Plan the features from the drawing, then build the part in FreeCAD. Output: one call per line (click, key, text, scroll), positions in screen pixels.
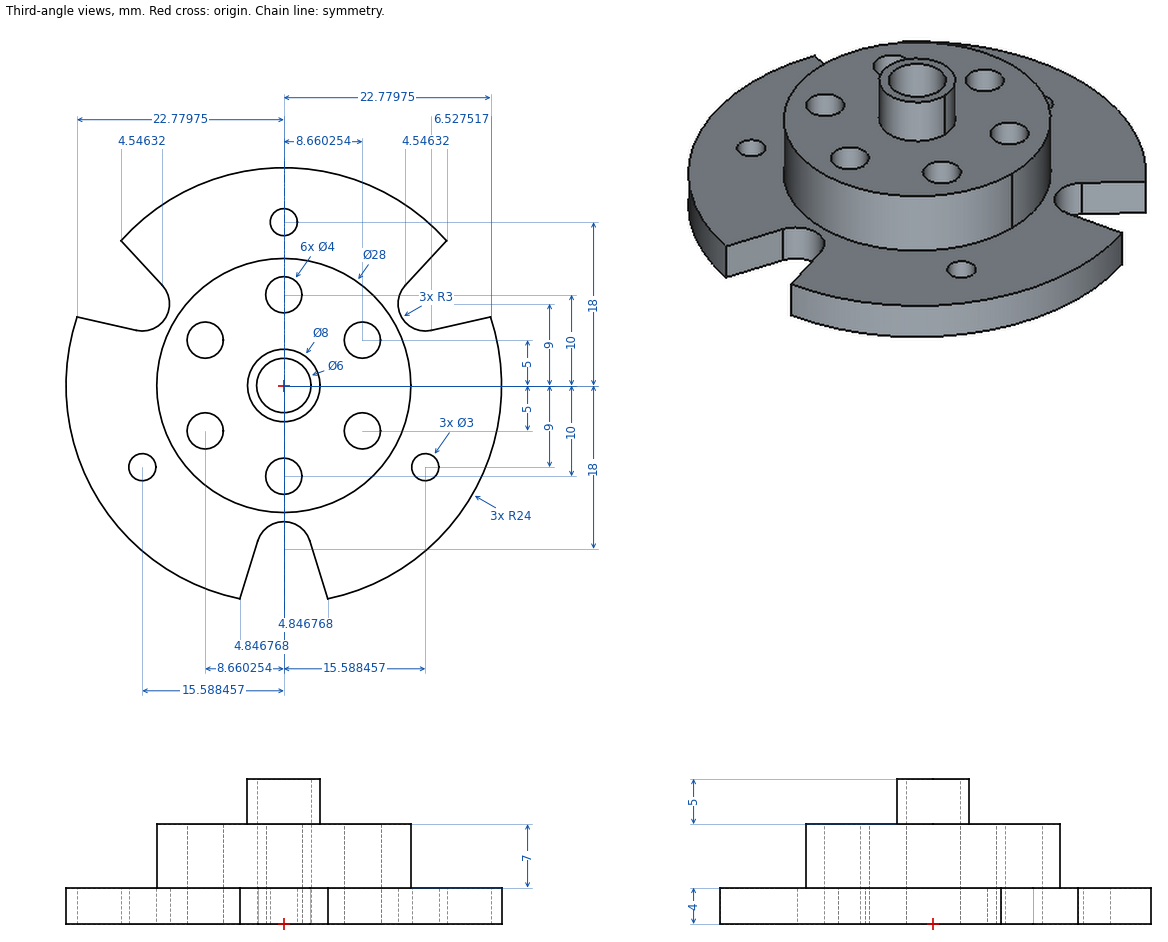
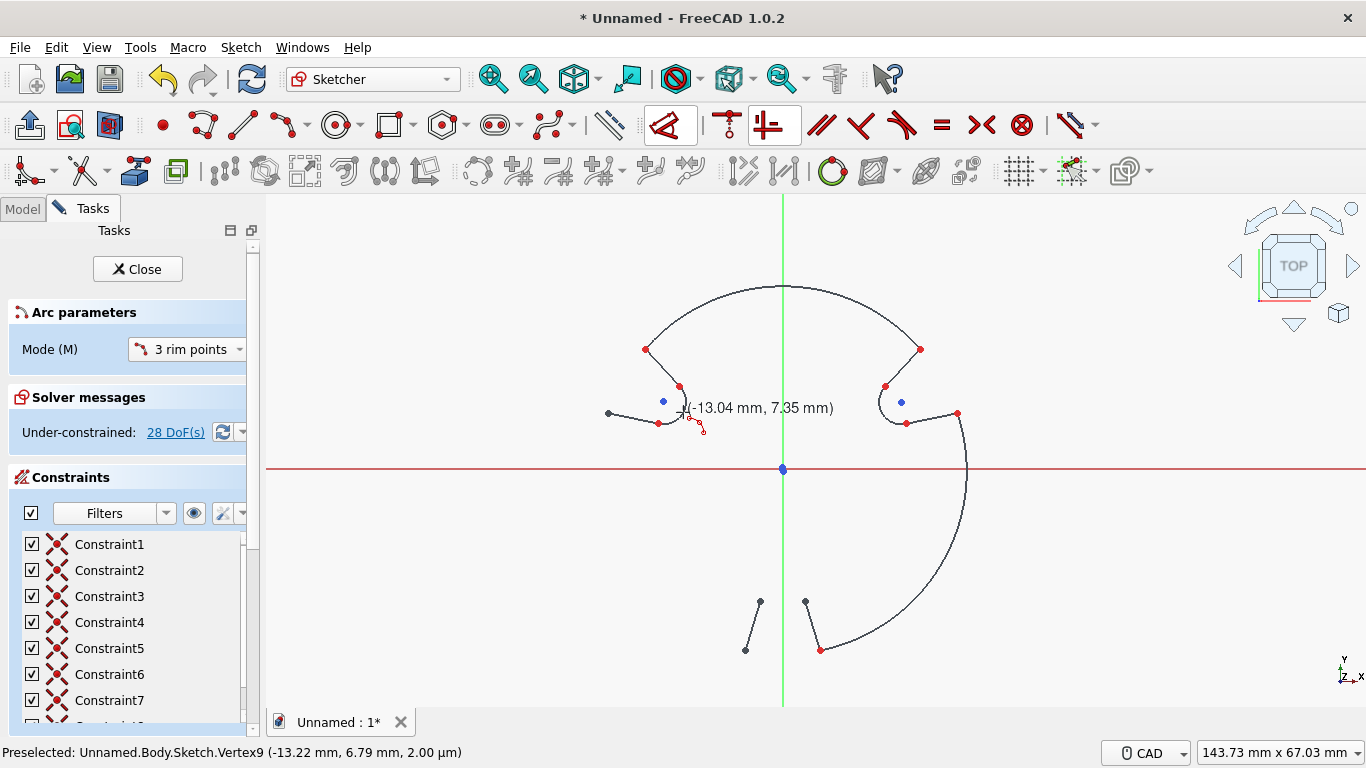
click(608, 413)
click(745, 650)
click(624, 561)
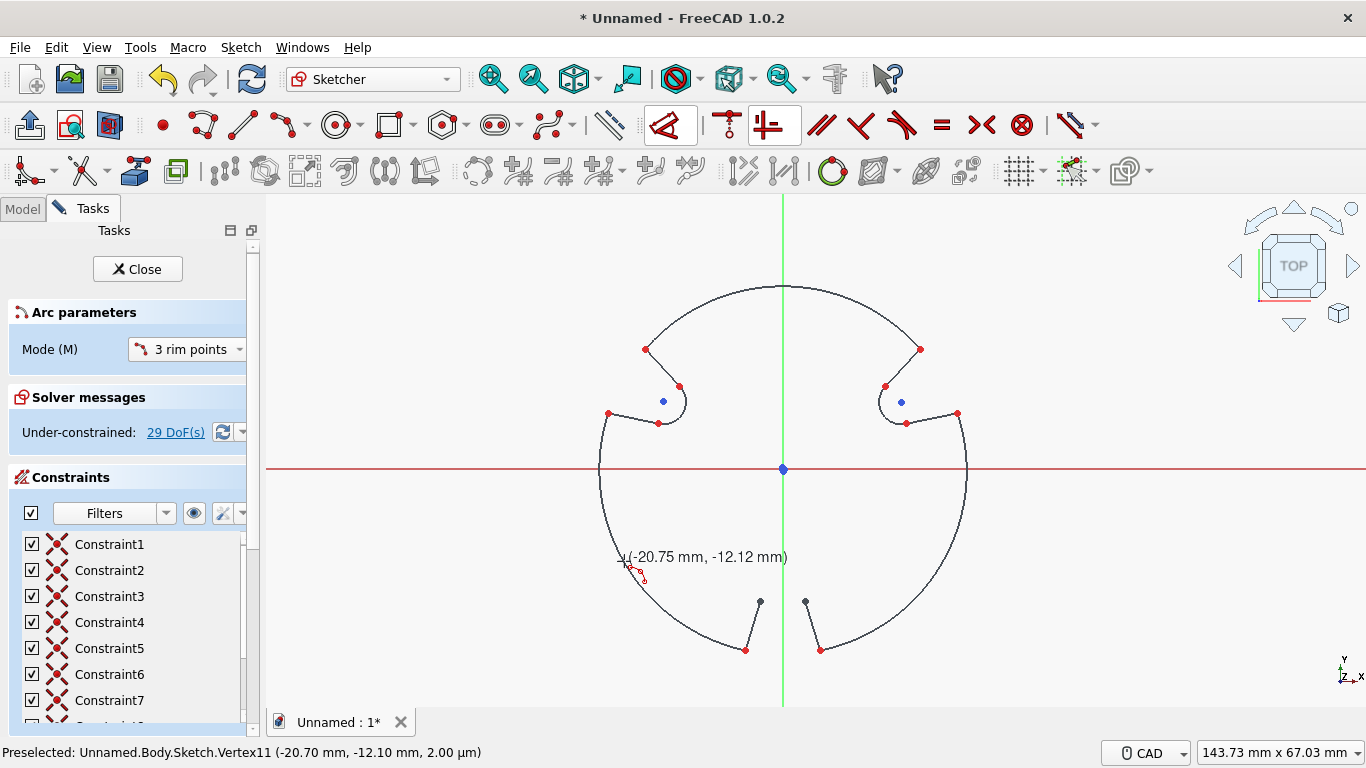
click(760, 601)
click(805, 601)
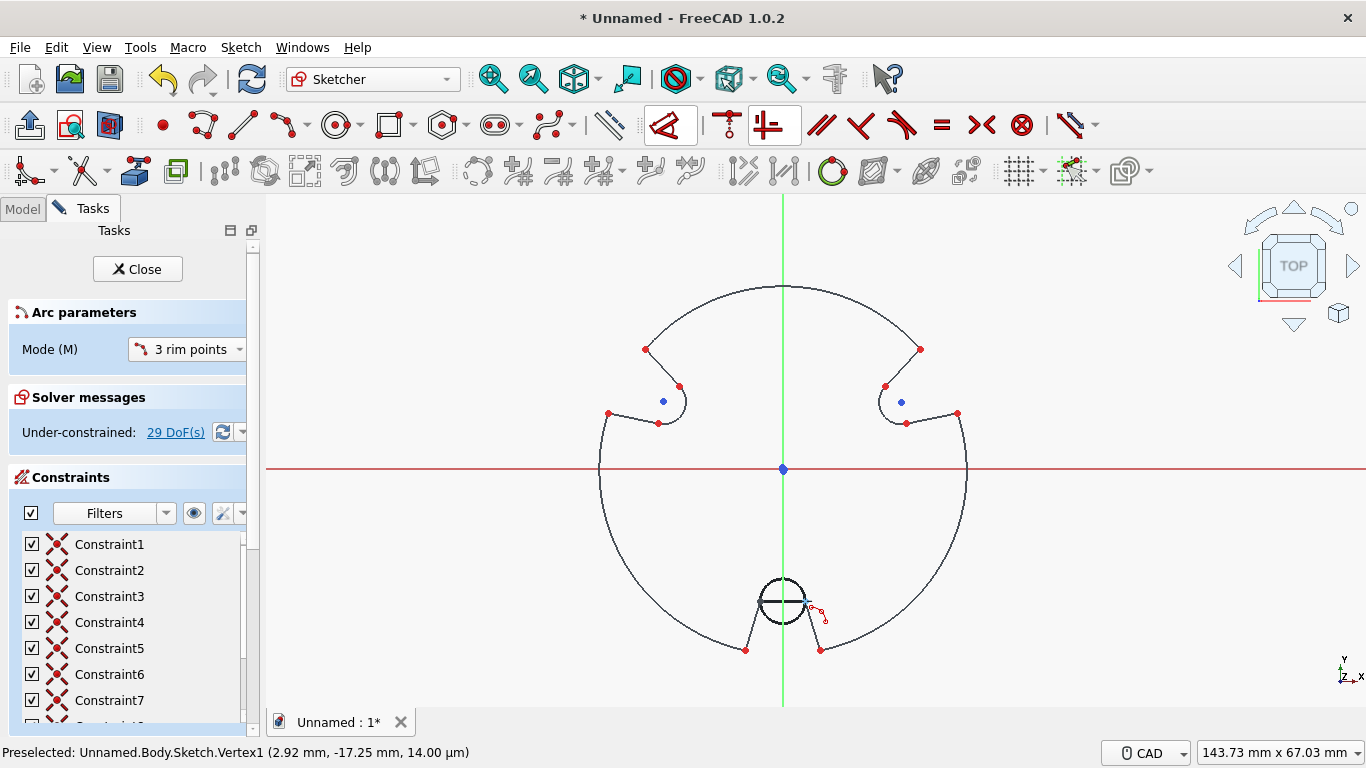
scroll(794, 587, up, 2)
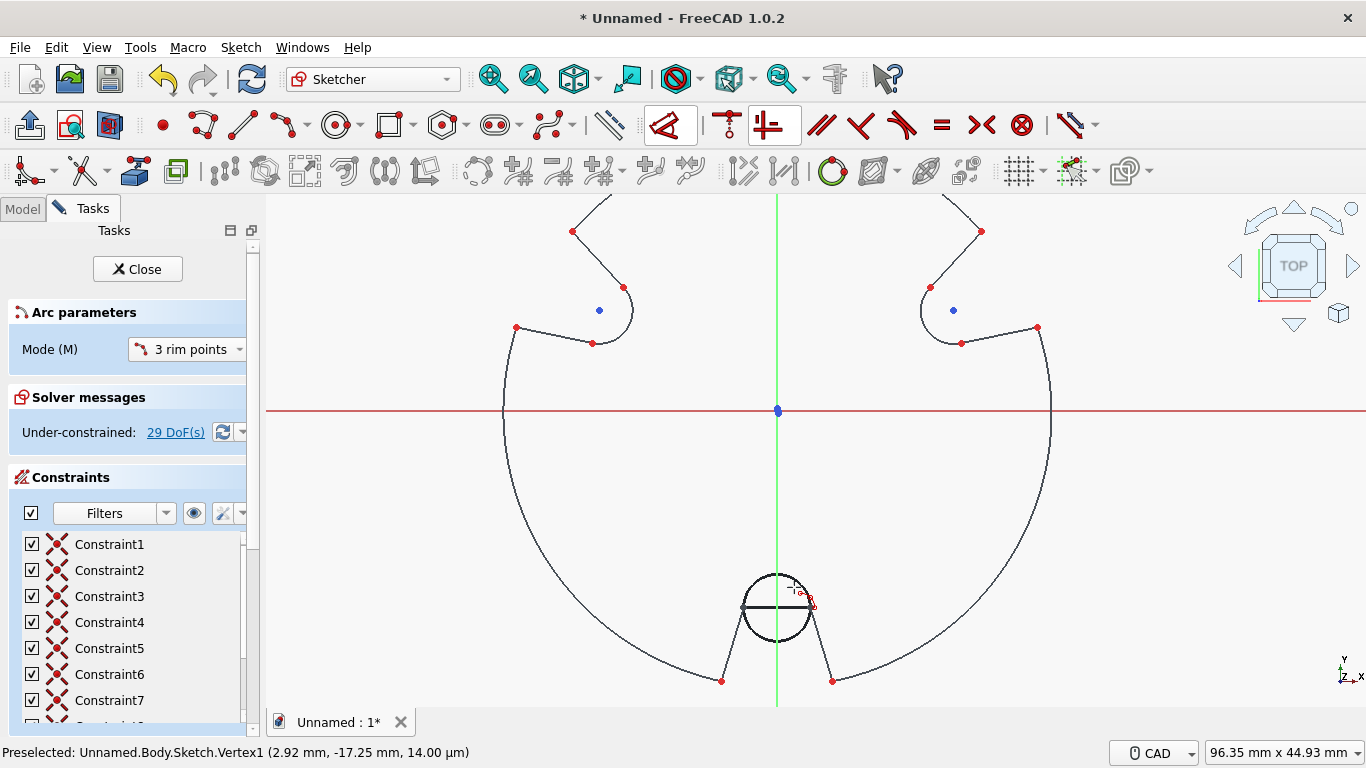
click(794, 587)
key(Escape)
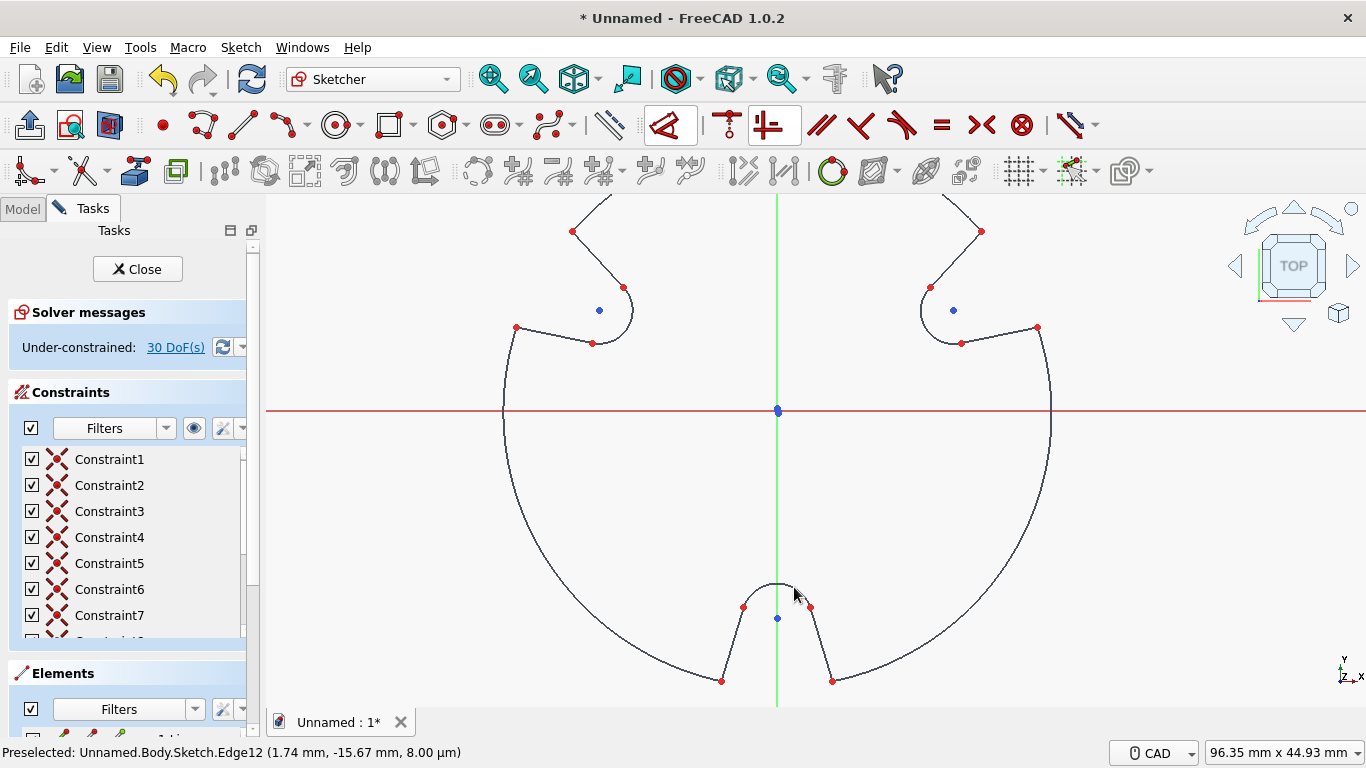
click(817, 630)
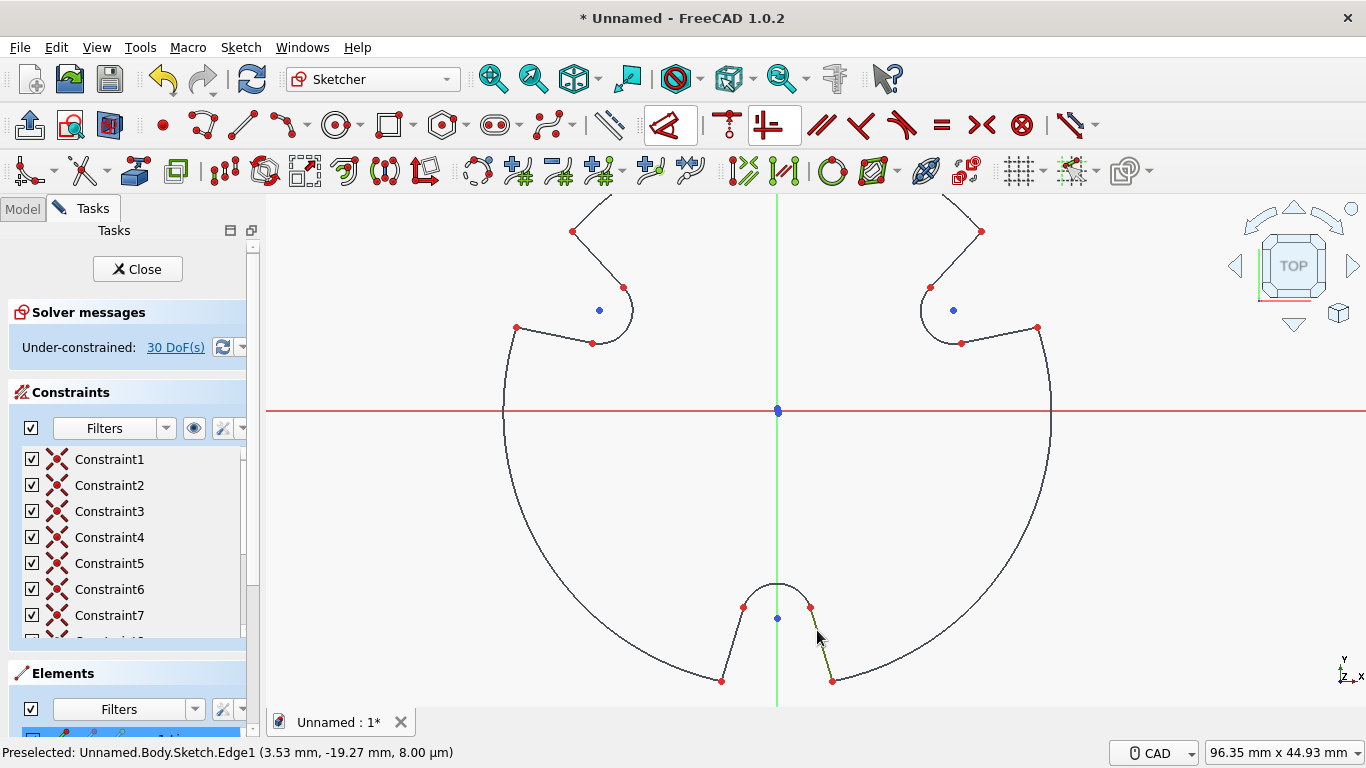
click(794, 588)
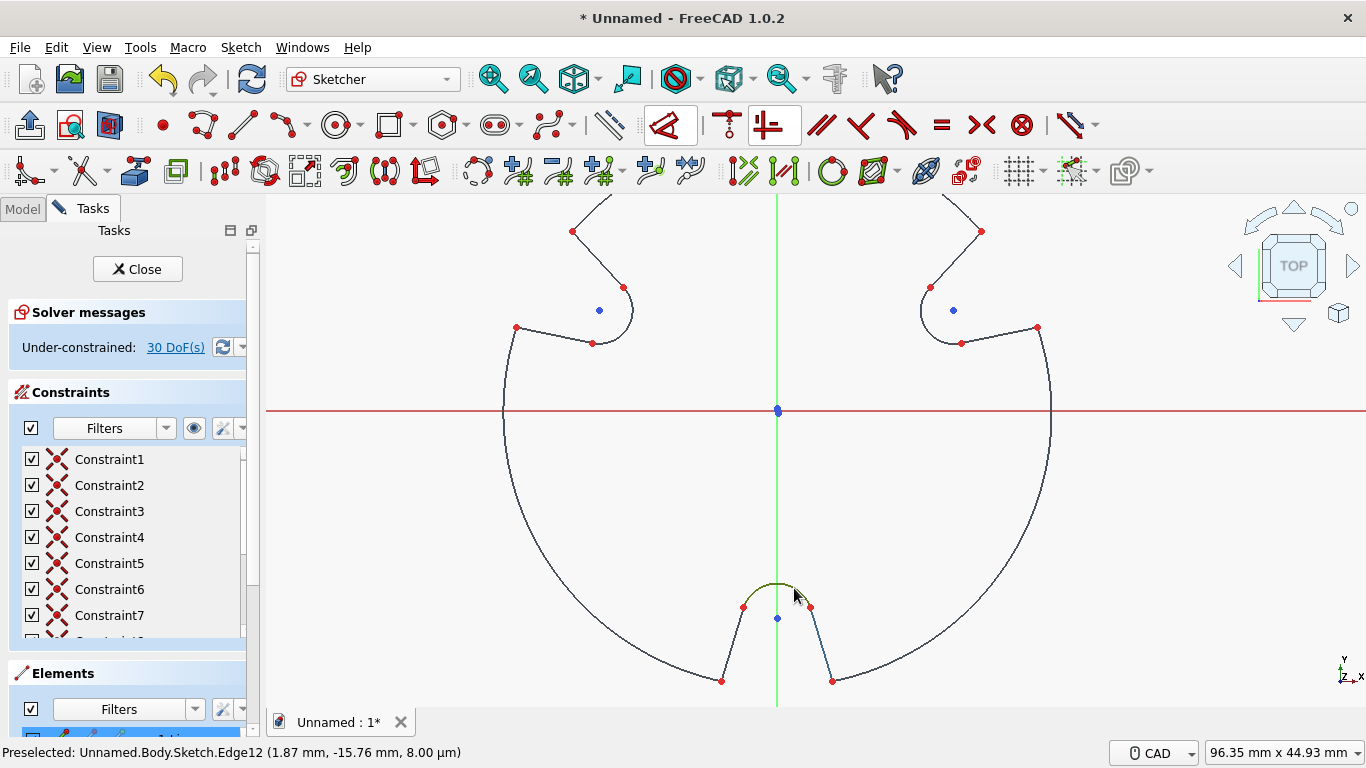
key(t)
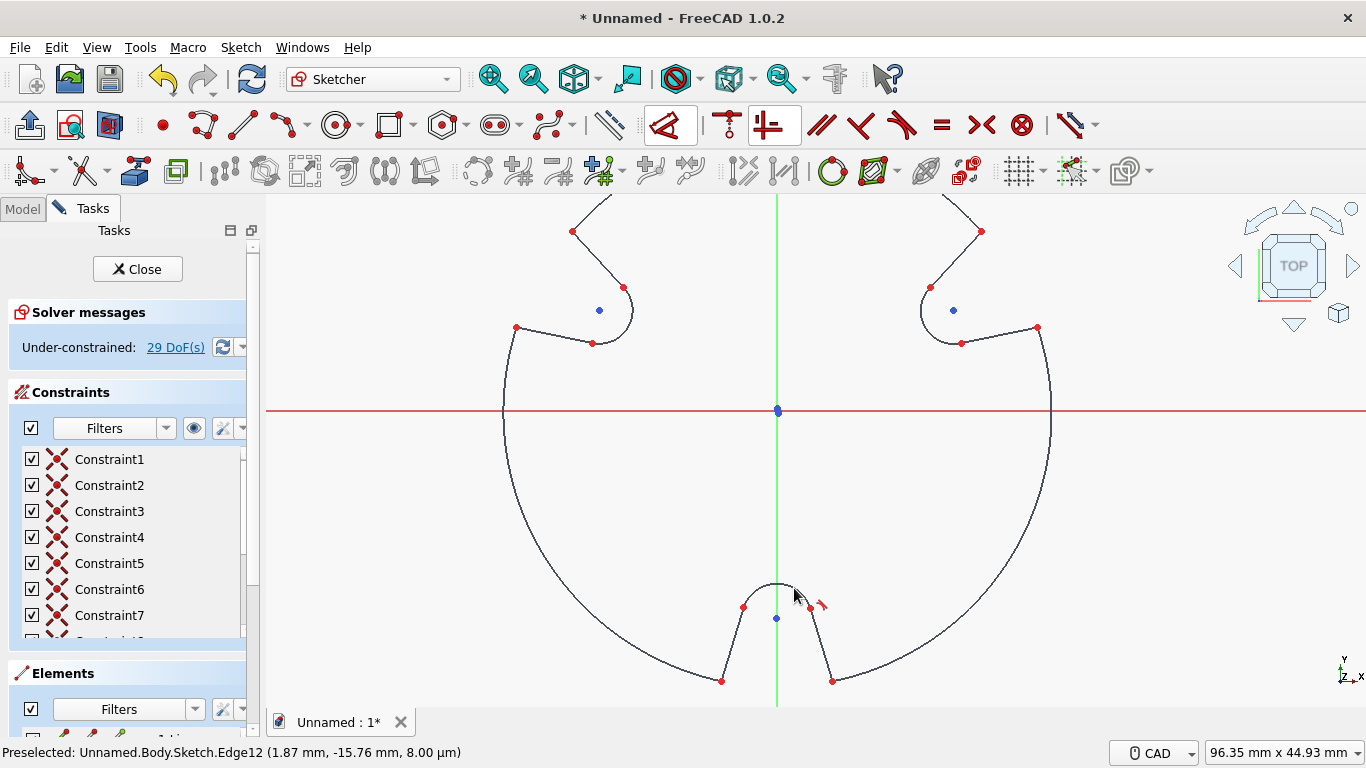
click(1015, 332)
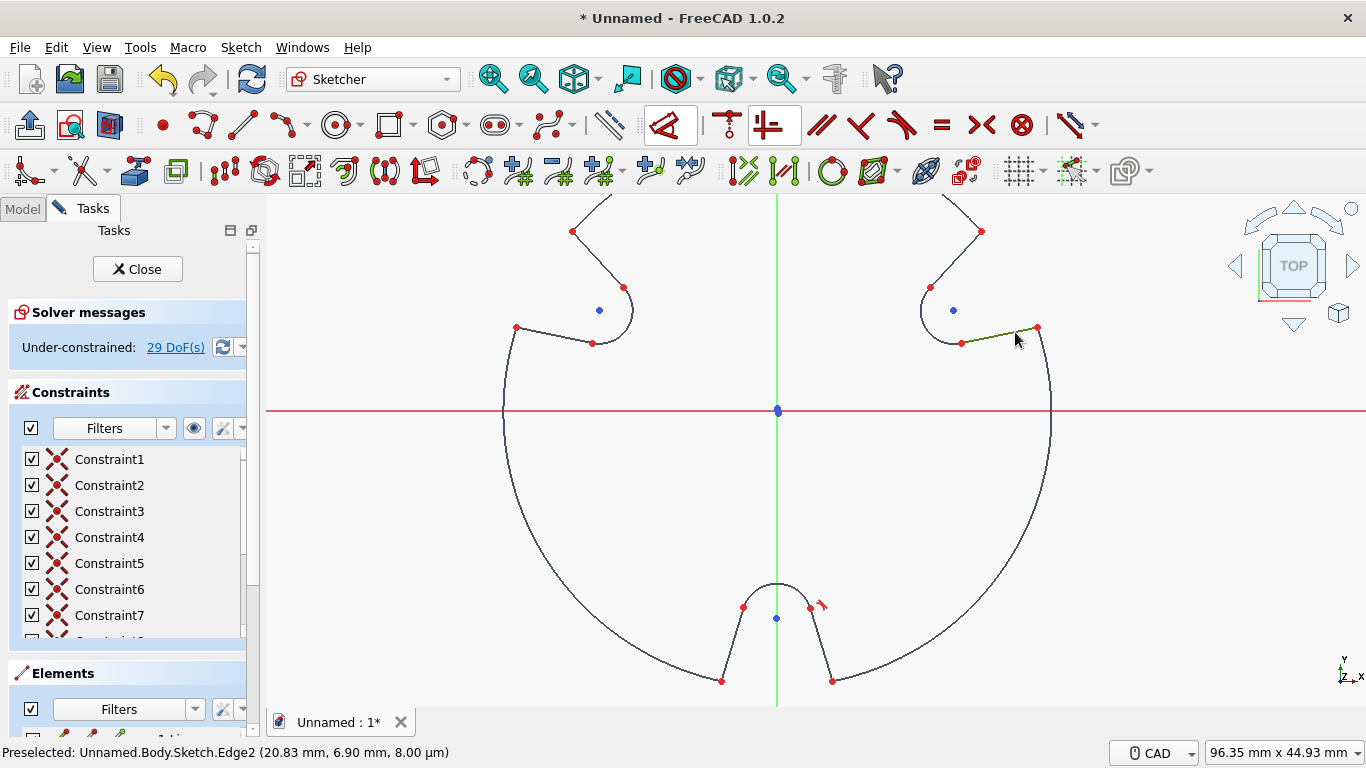
click(921, 311)